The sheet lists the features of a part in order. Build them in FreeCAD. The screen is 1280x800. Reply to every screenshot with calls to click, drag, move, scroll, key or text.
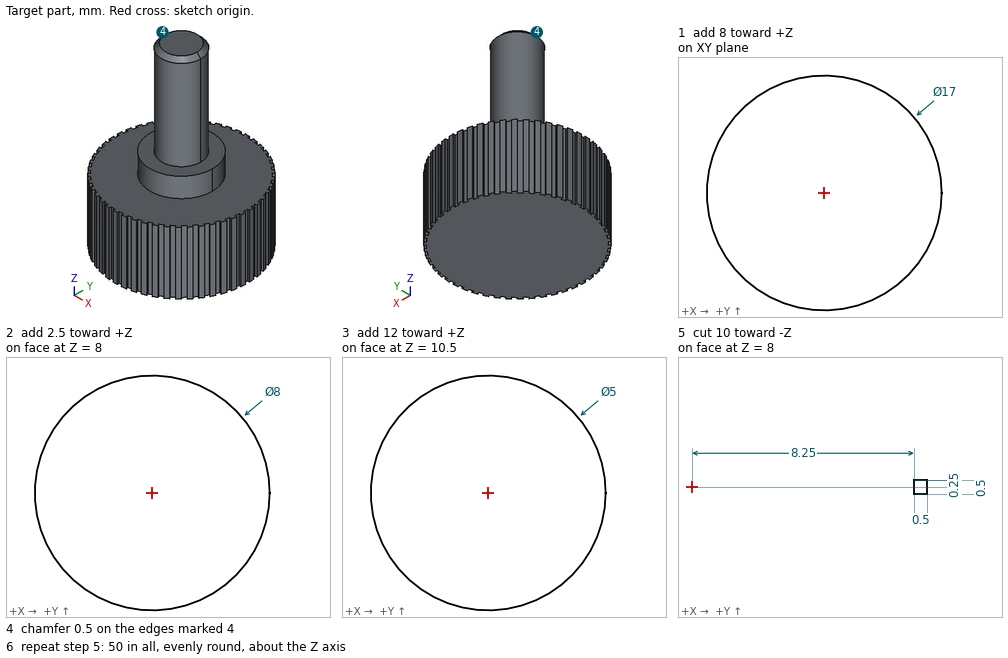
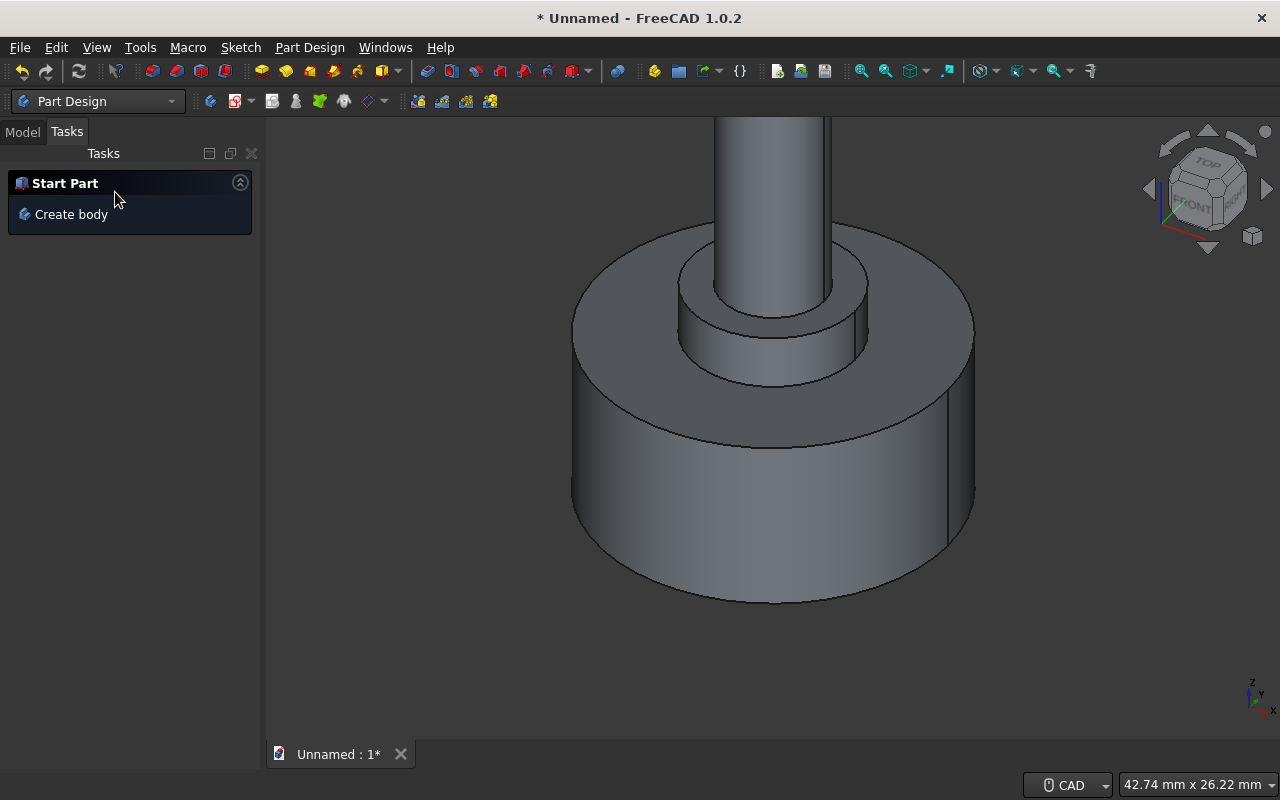
key(v)
key(f)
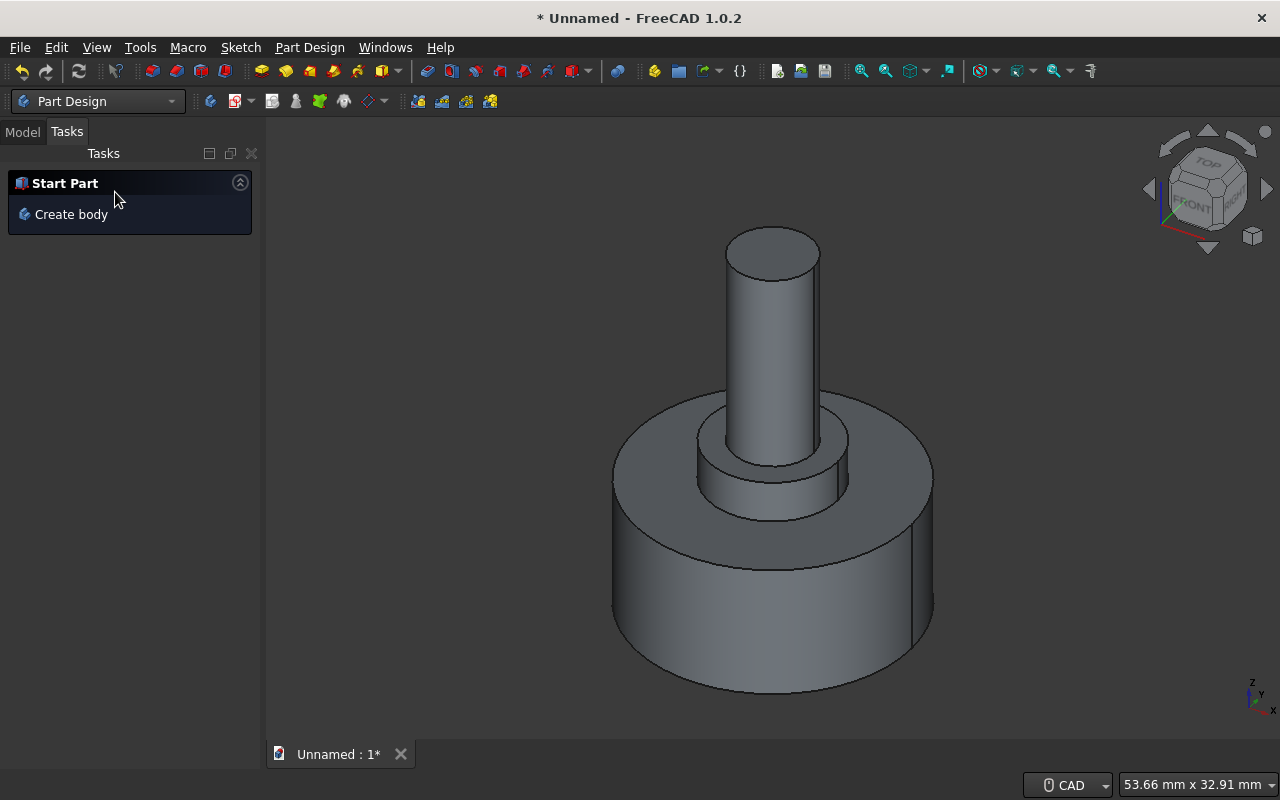
click(726, 256)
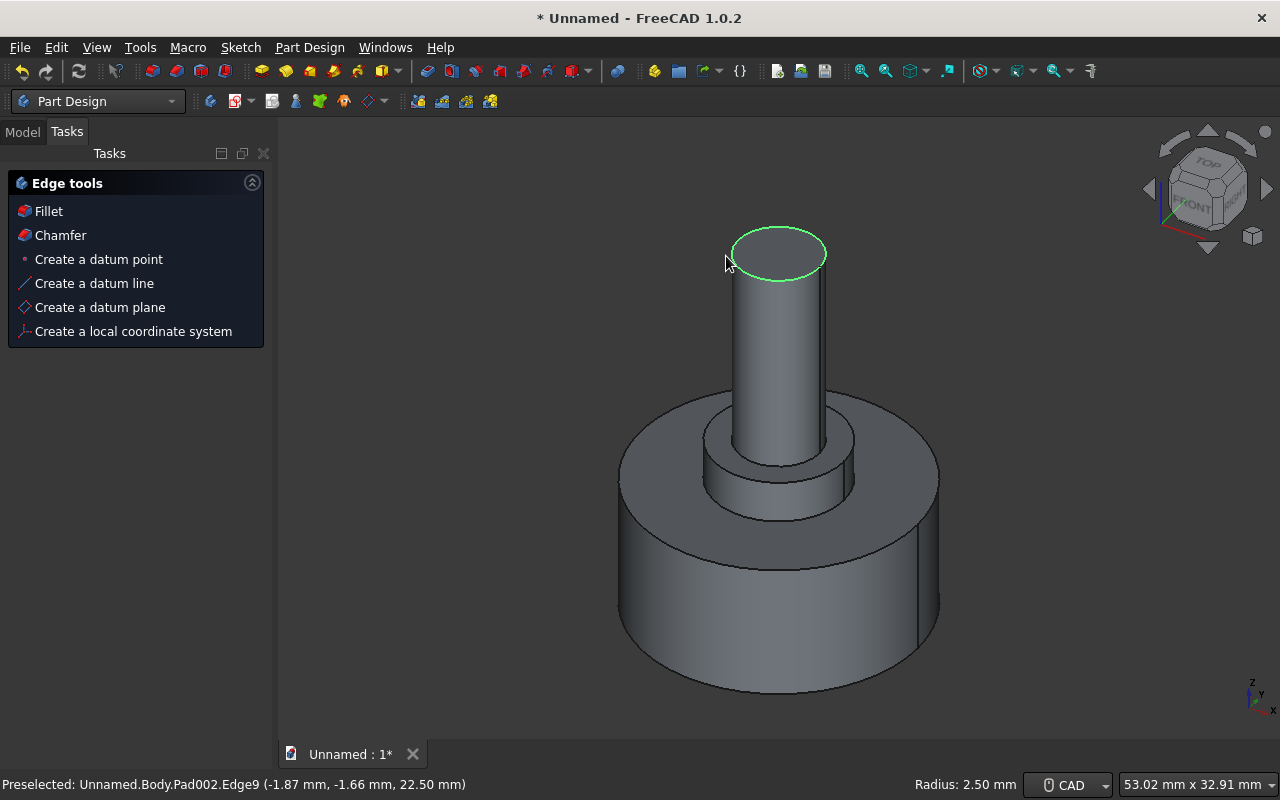
click(178, 72)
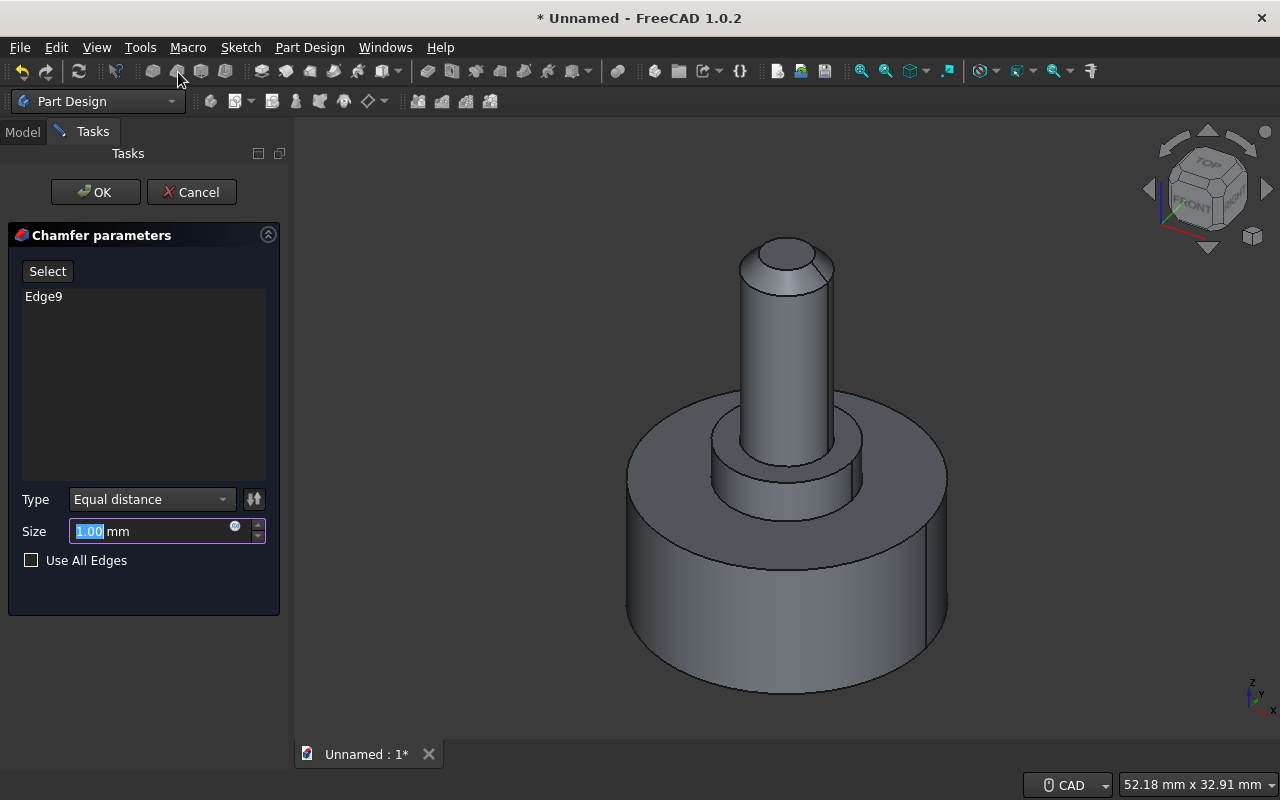
text(0.5)
key(Tab)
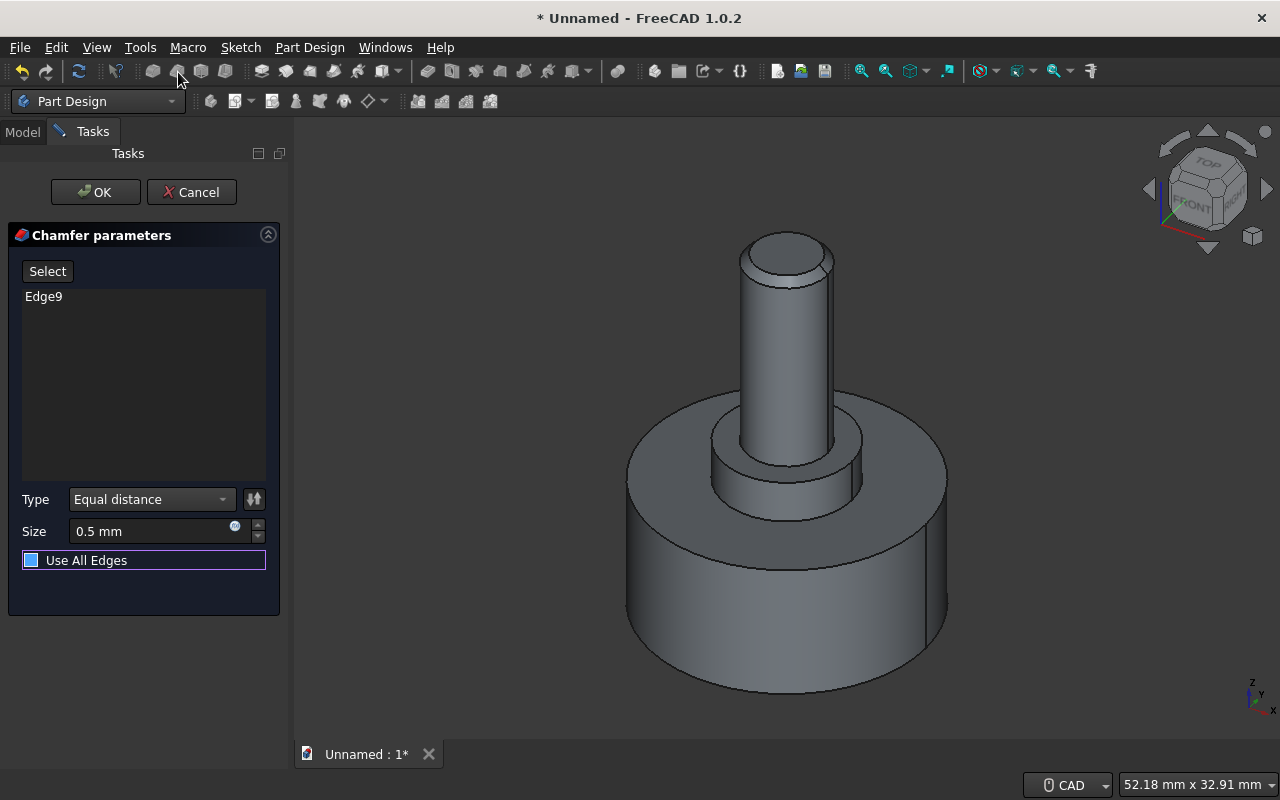
click(96, 192)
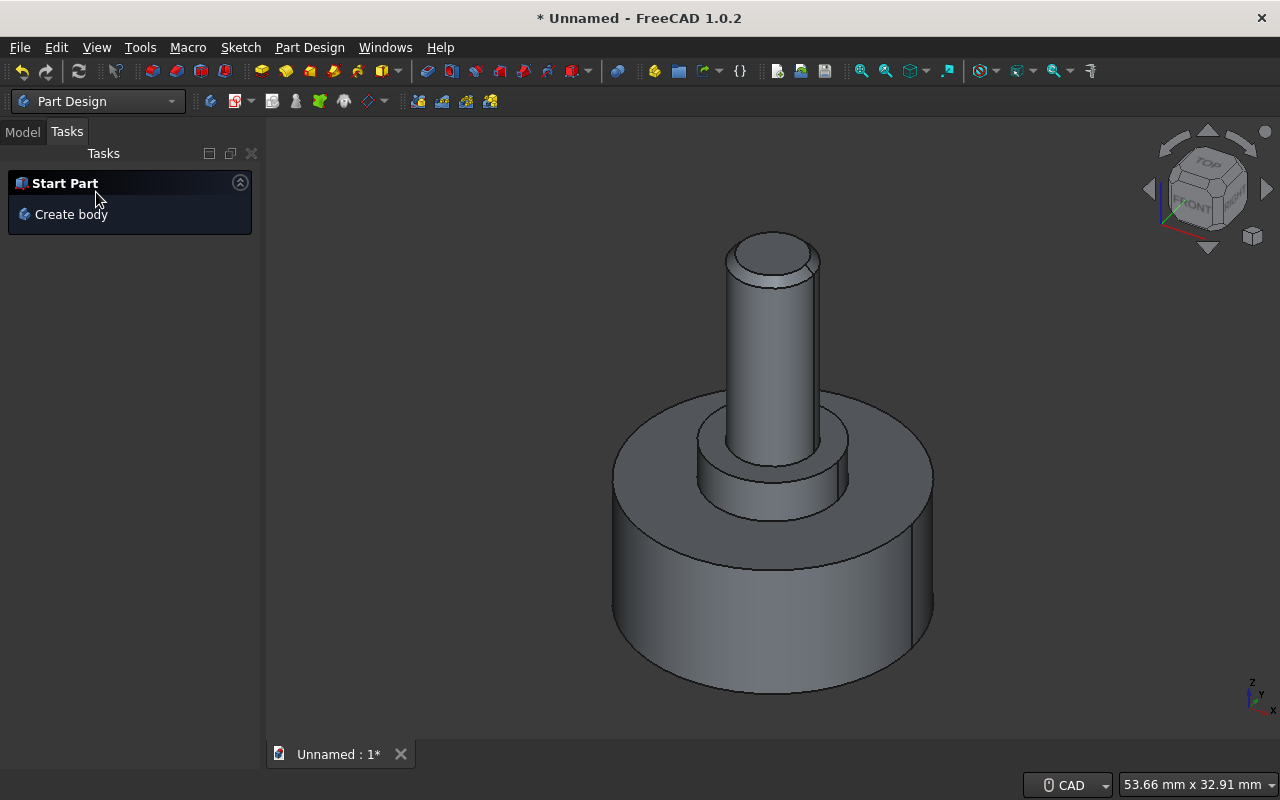
click(806, 549)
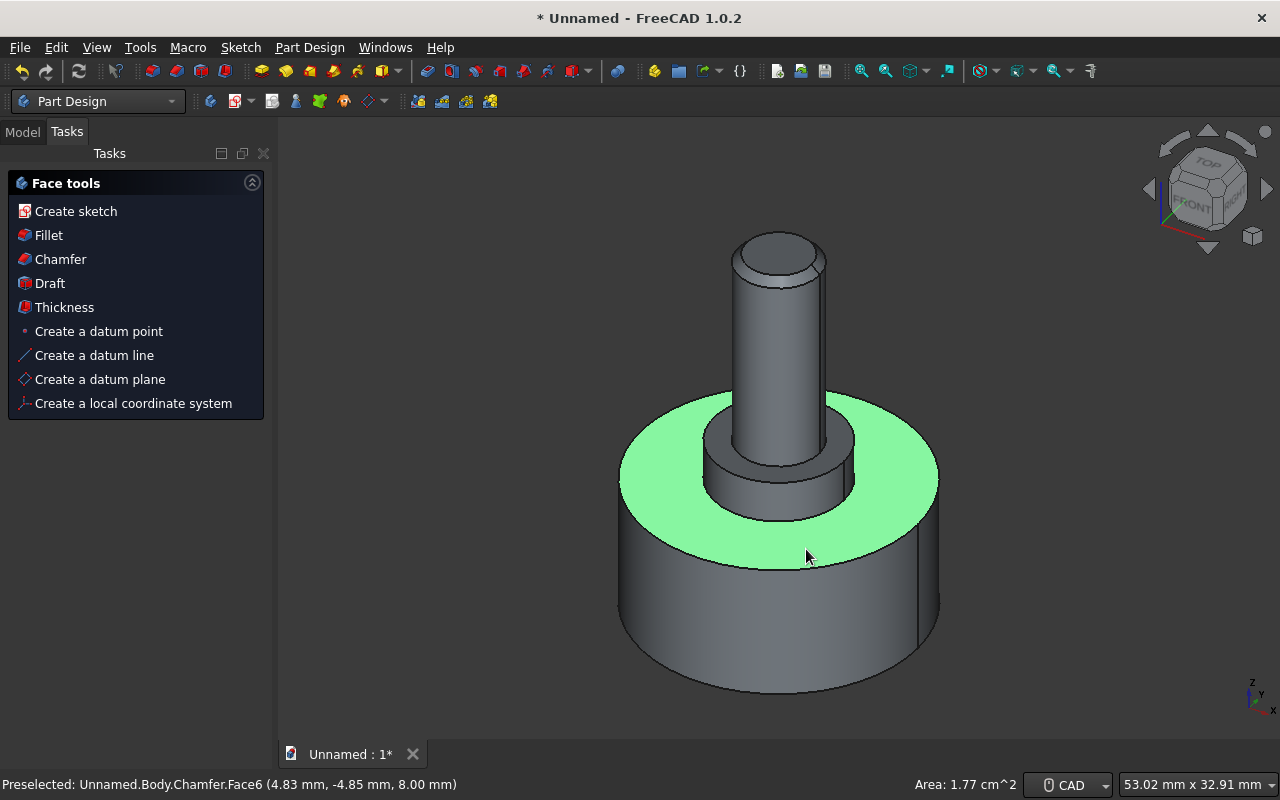
click(236, 102)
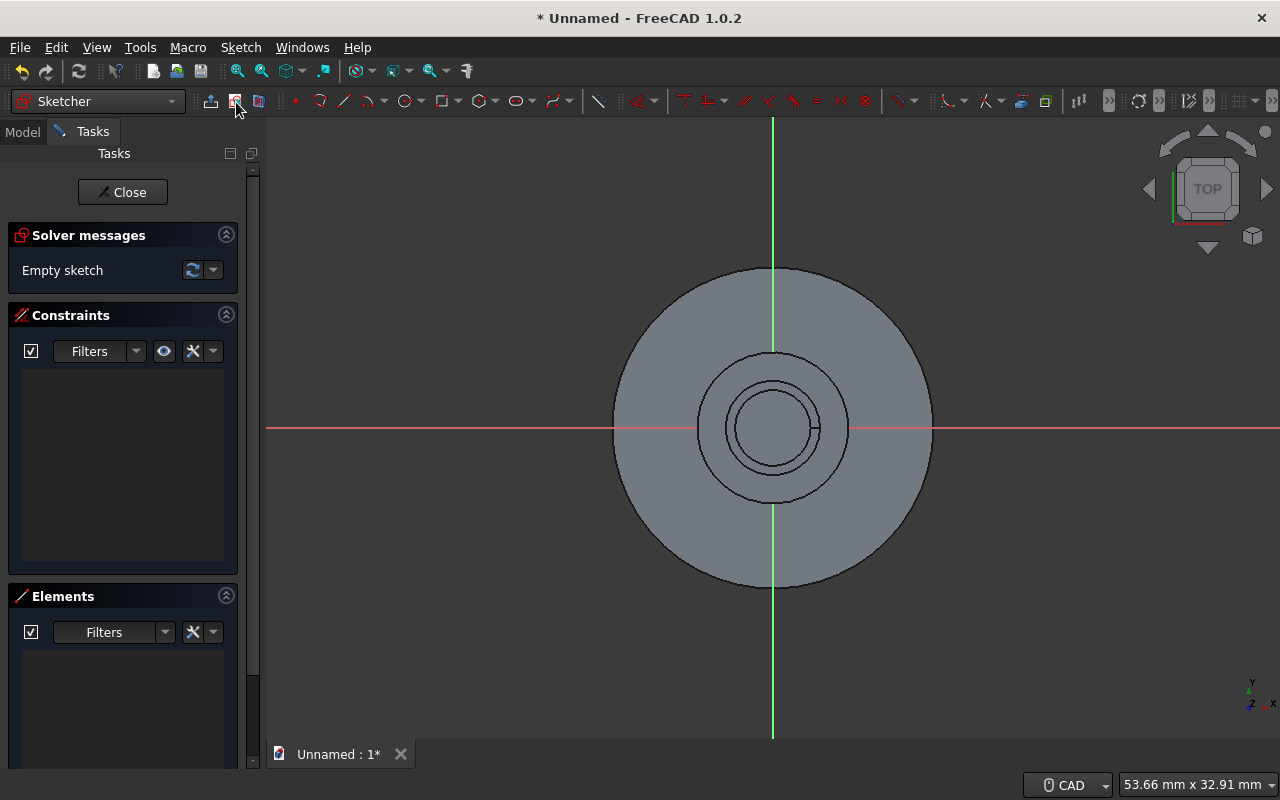
key(q)
key(s)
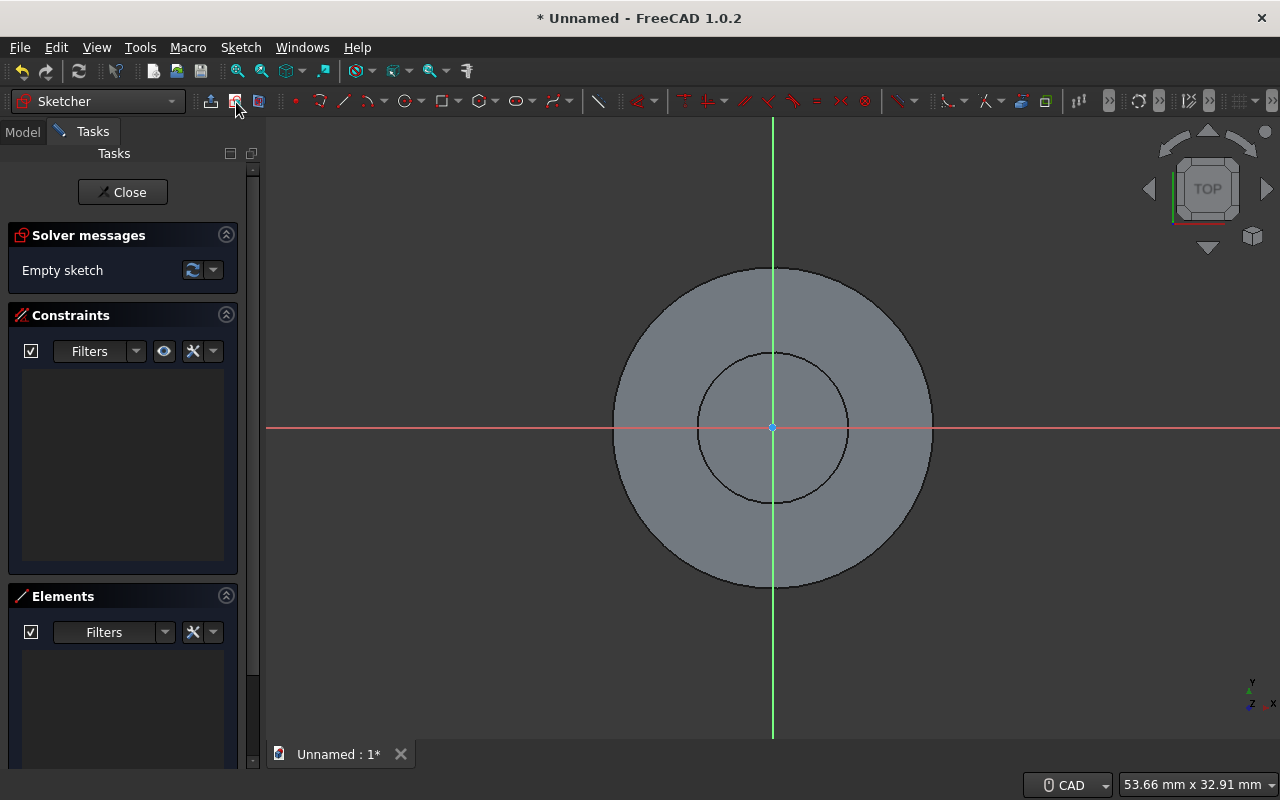
scroll(945, 428, up, 15)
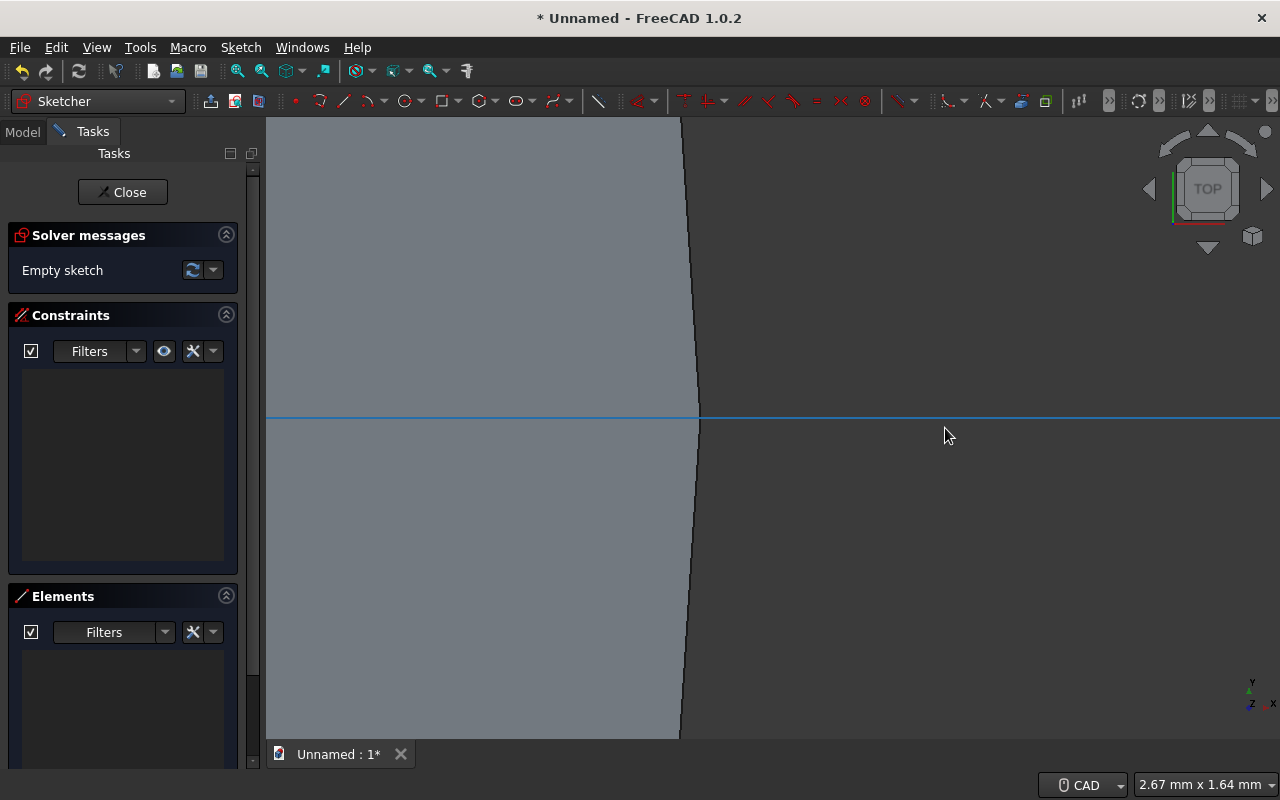
scroll(697, 411, up, 4)